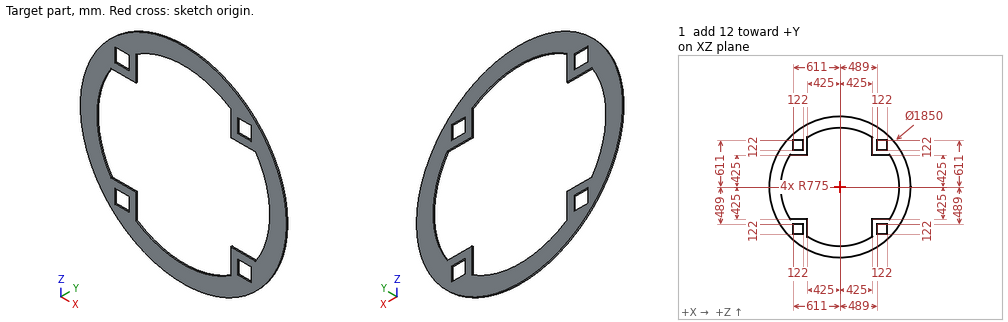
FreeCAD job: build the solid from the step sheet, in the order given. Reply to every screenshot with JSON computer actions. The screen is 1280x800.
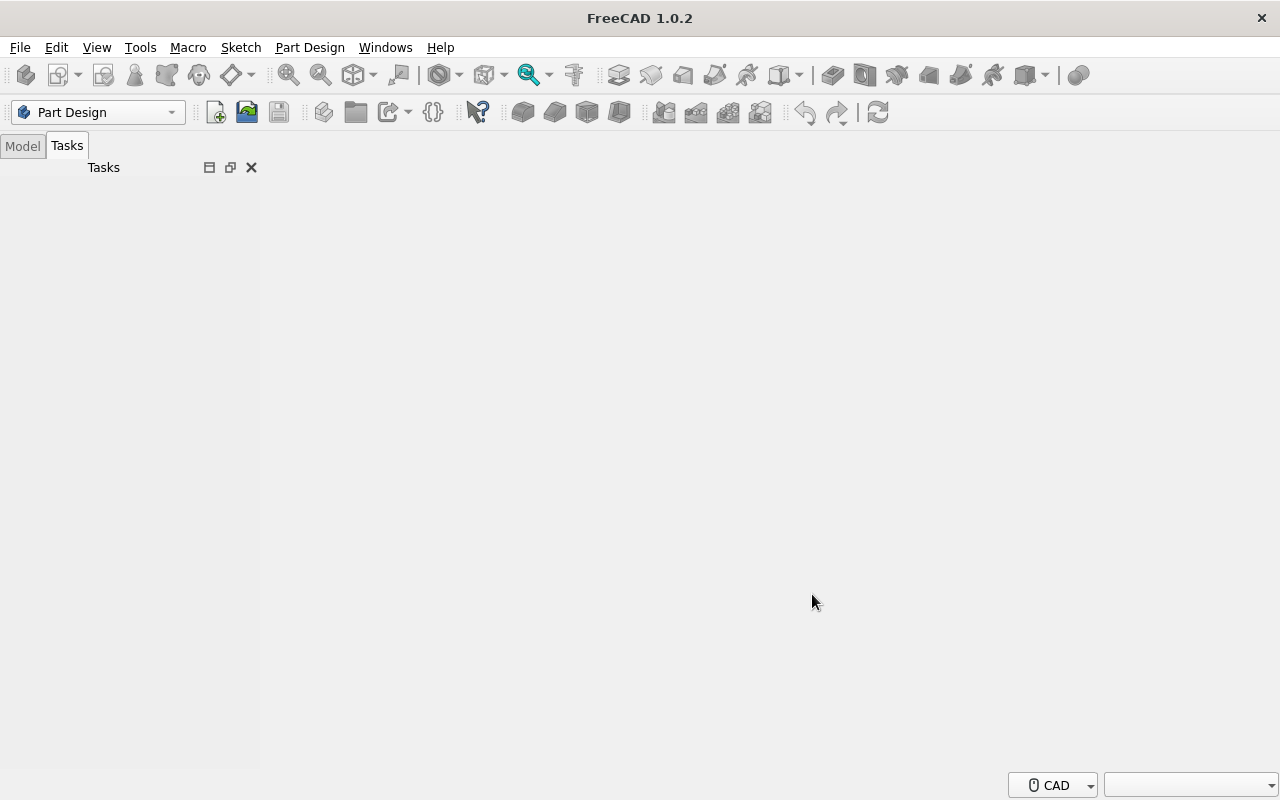
{"action": "left_click", "coordinate": [216, 112]}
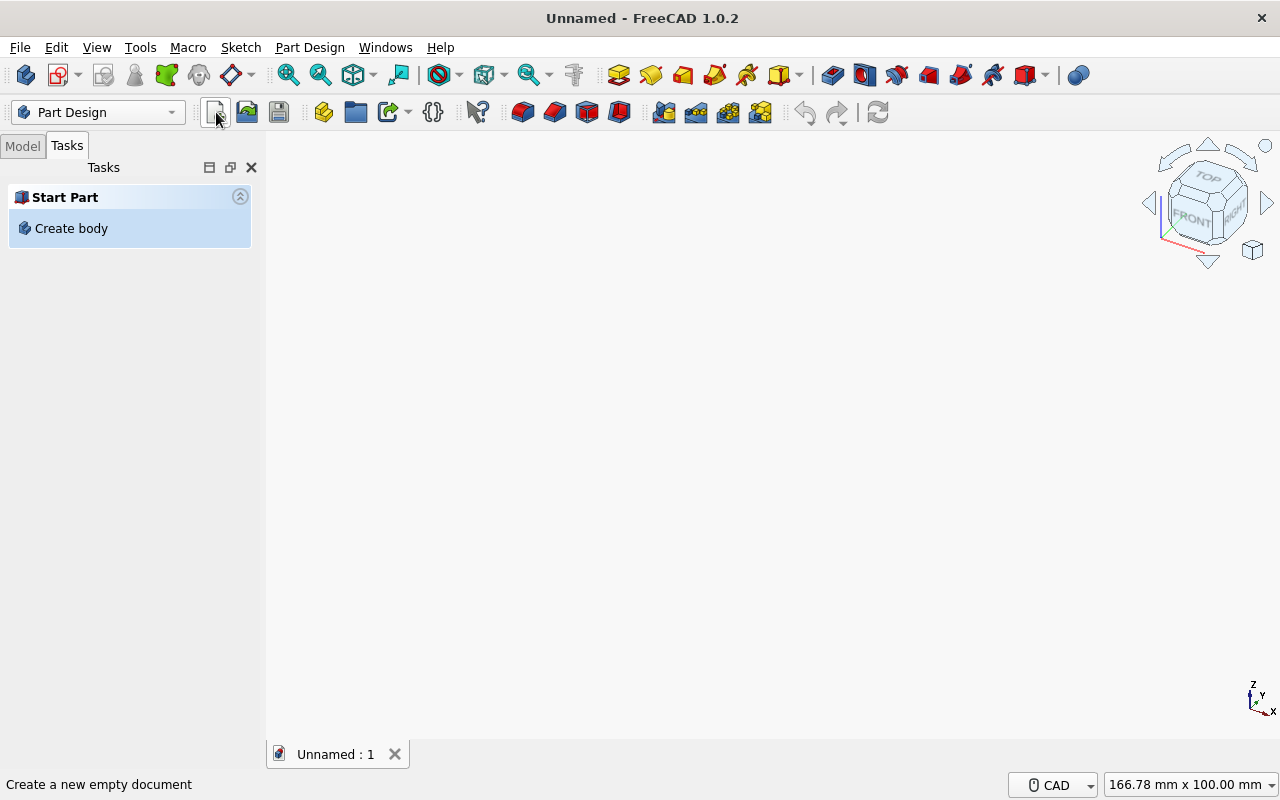
{"action": "left_click", "coordinate": [58, 76]}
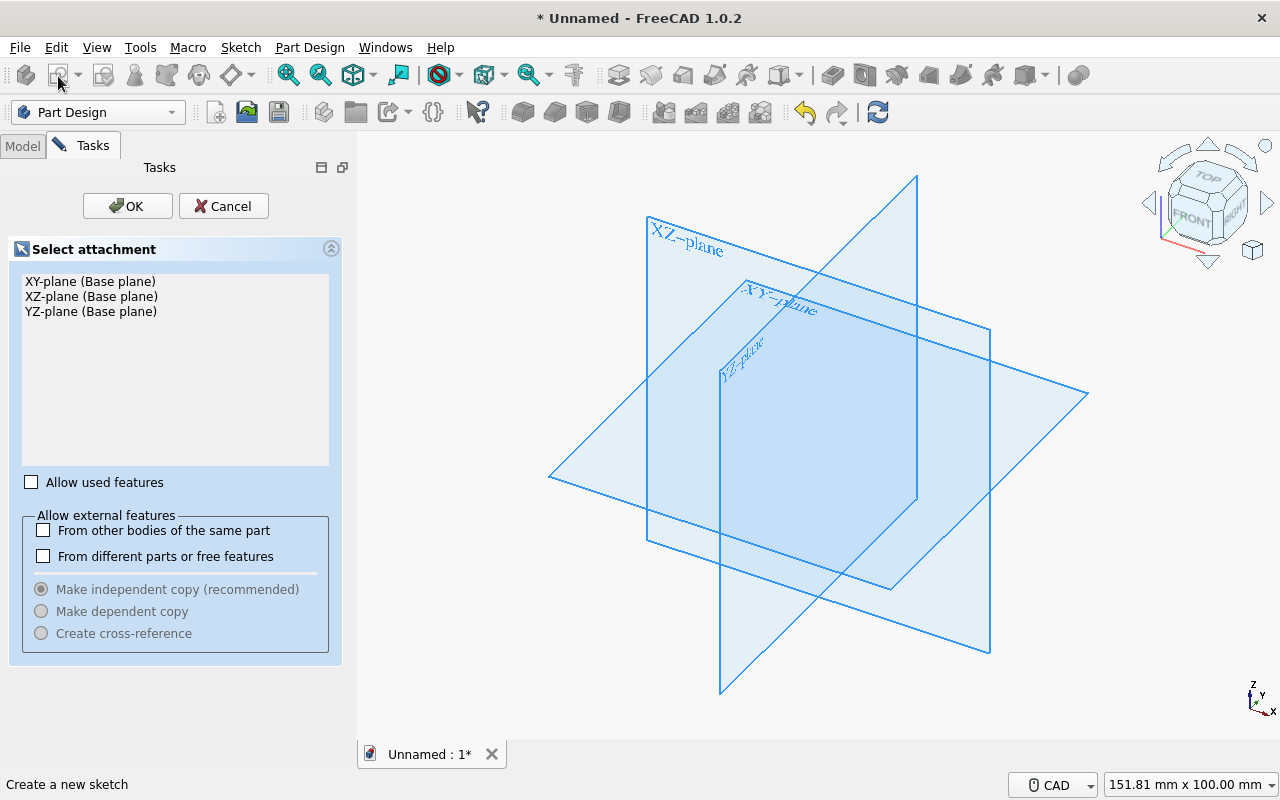
{"action": "left_click", "coordinate": [82, 296]}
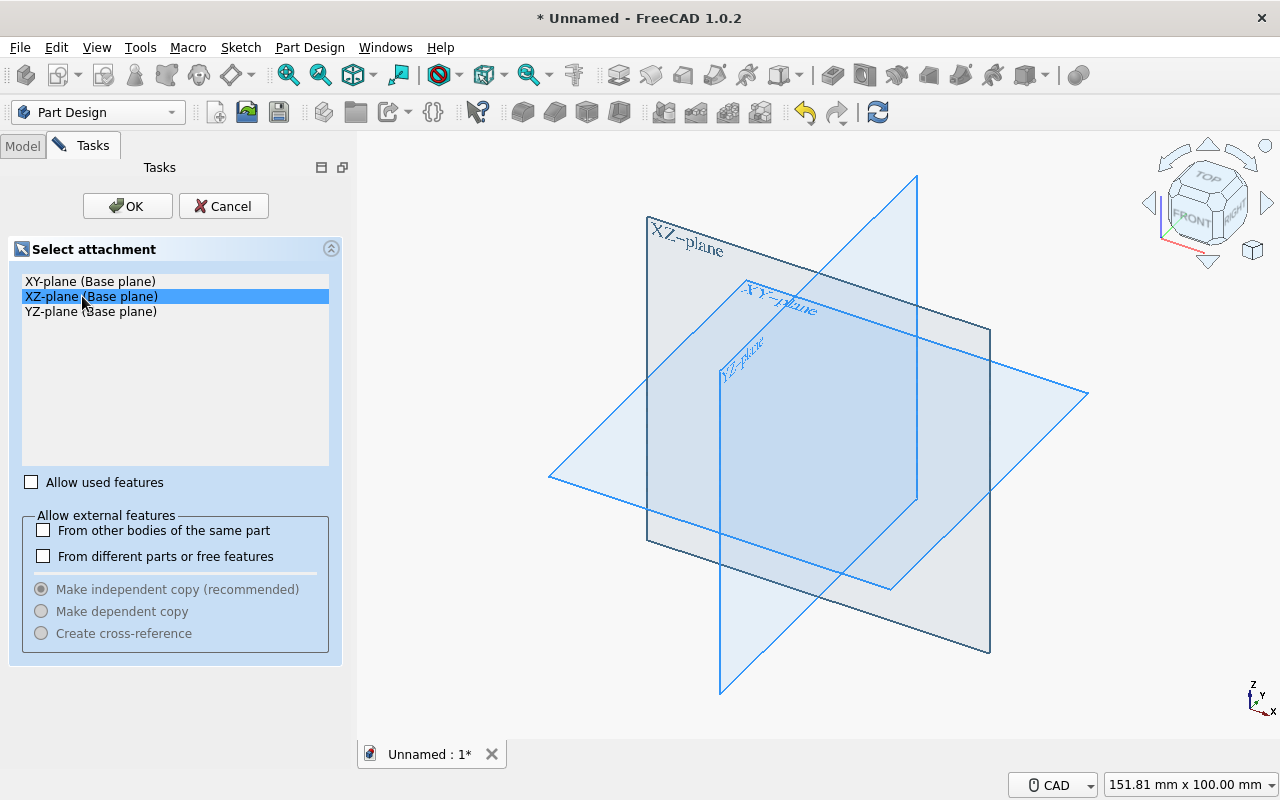
{"action": "left_click", "coordinate": [128, 206]}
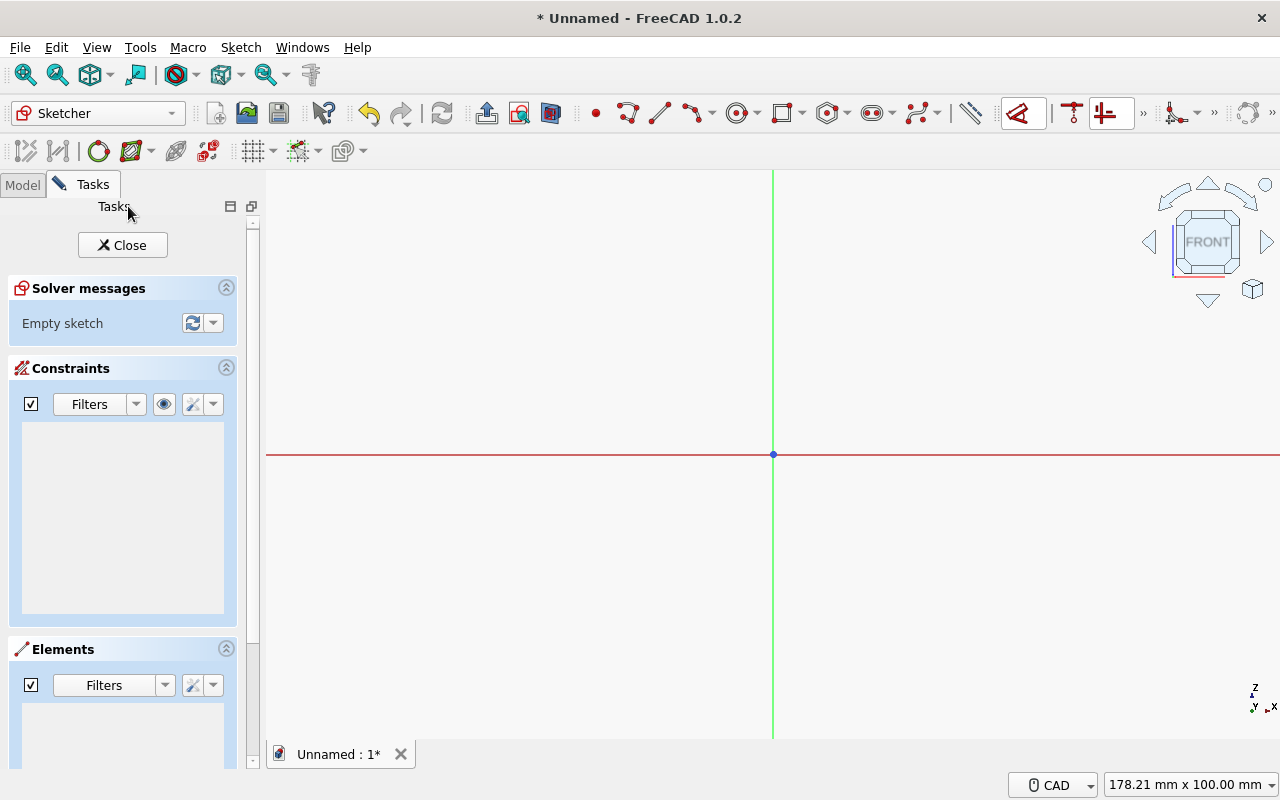
{"action": "scroll", "coordinate": [702, 454], "scroll_direction": "down", "scroll_amount": 16}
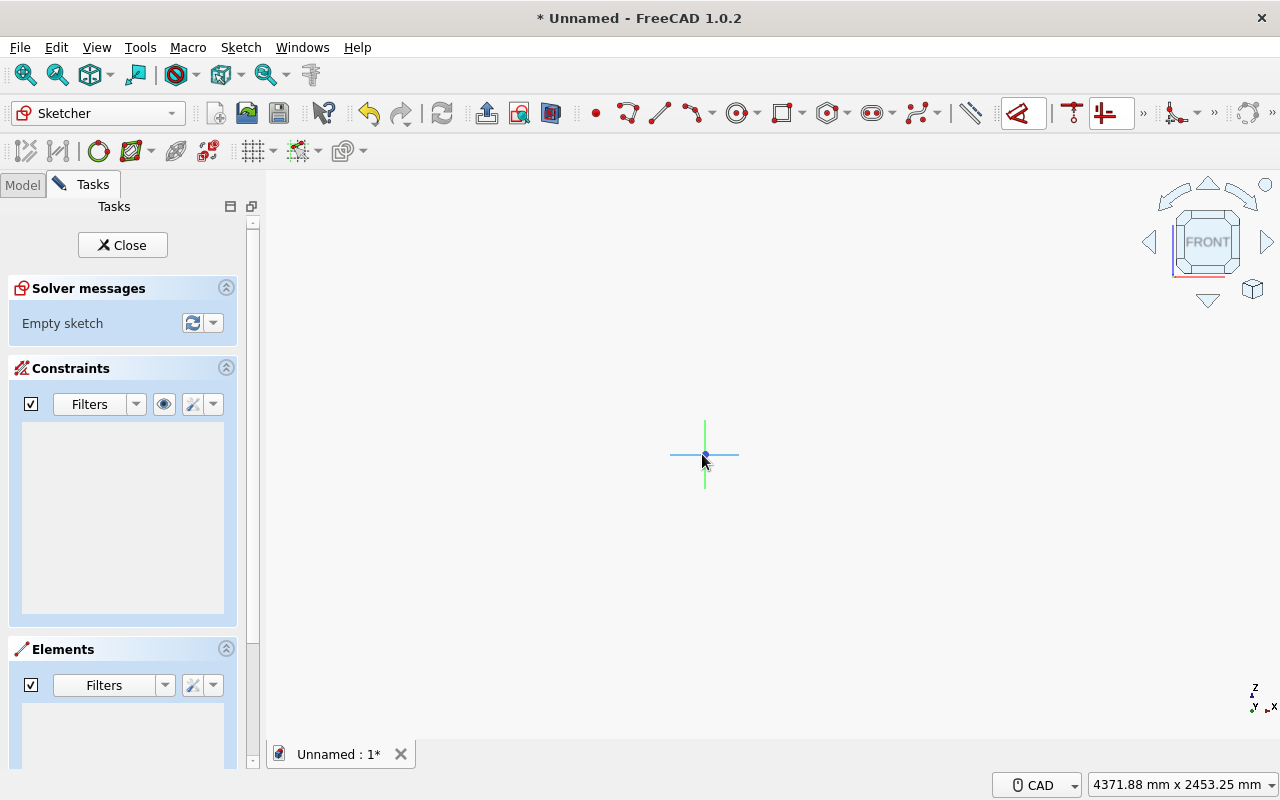
{"action": "left_click", "coordinate": [782, 114]}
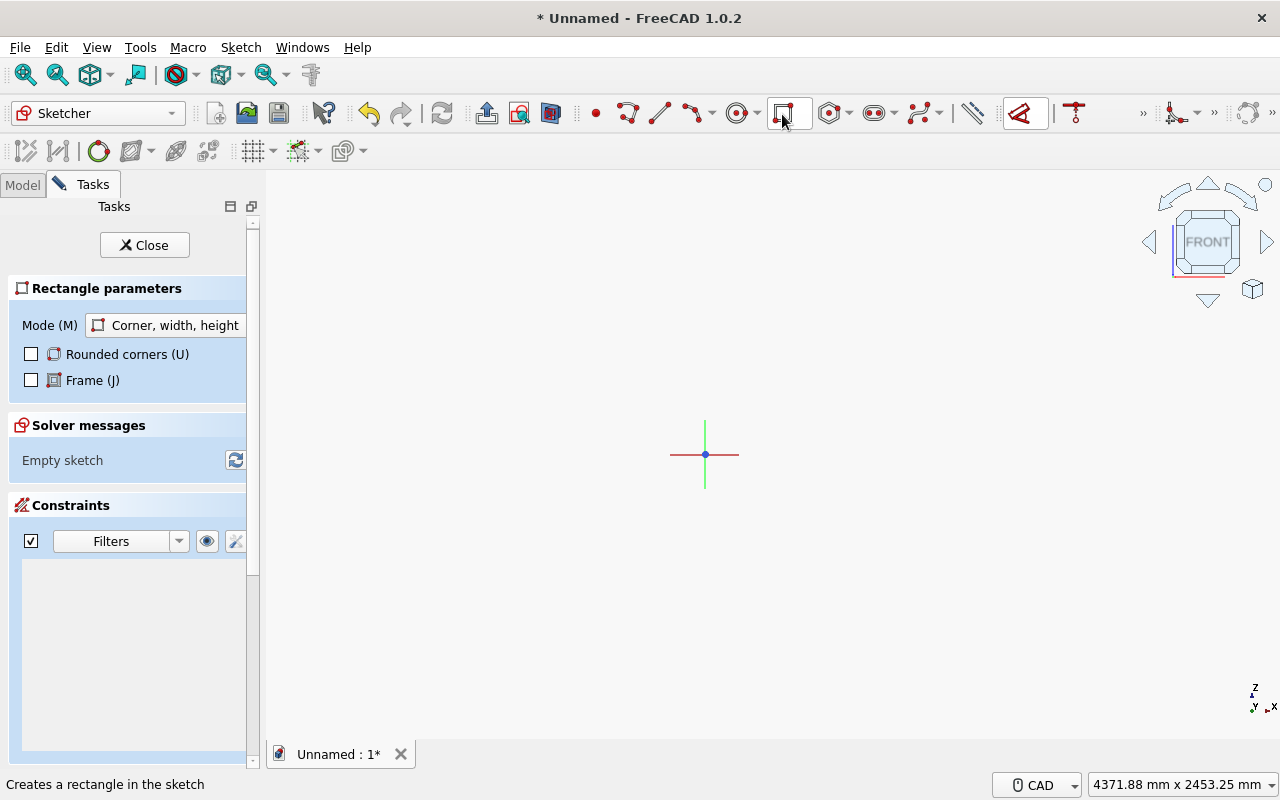
{"action": "left_click", "coordinate": [564, 568]}
{"action": "left_click", "coordinate": [592, 596]}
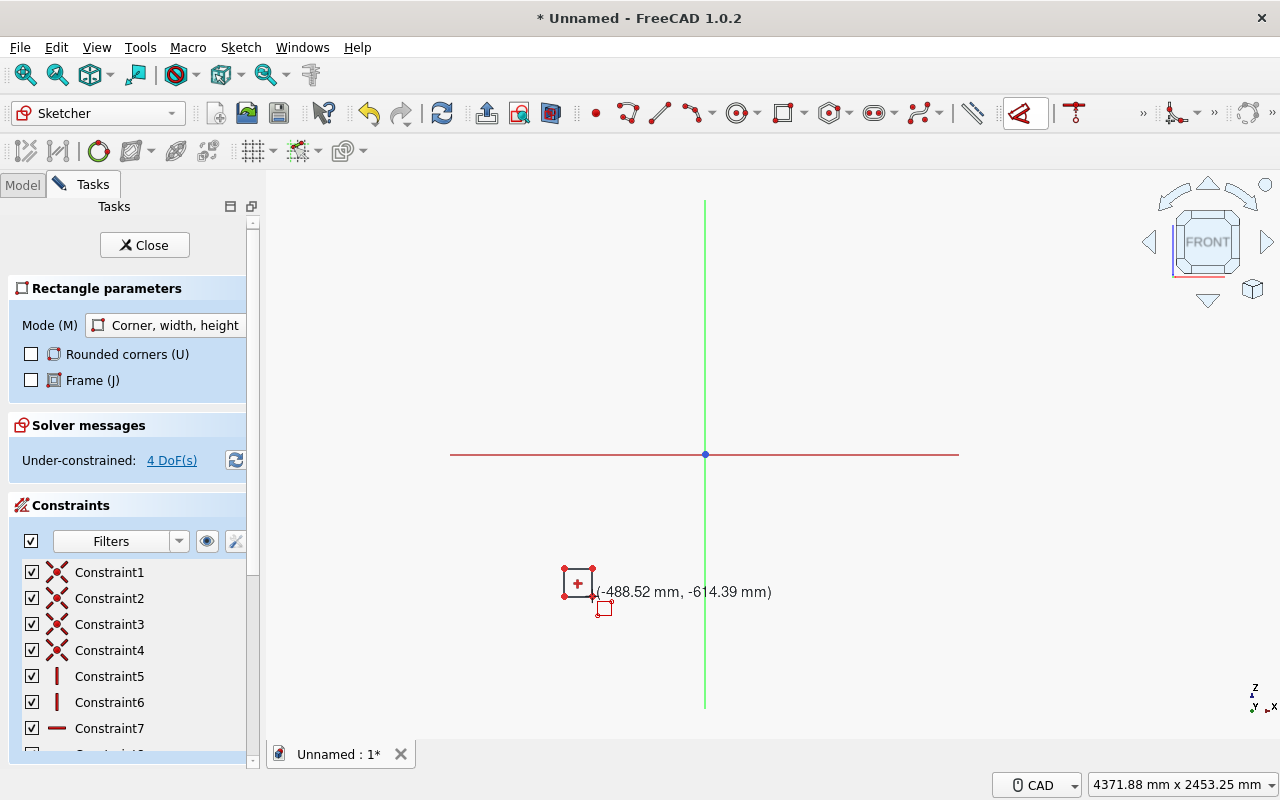
{"action": "left_click", "coordinate": [564, 313]}
{"action": "left_click", "coordinate": [592, 341]}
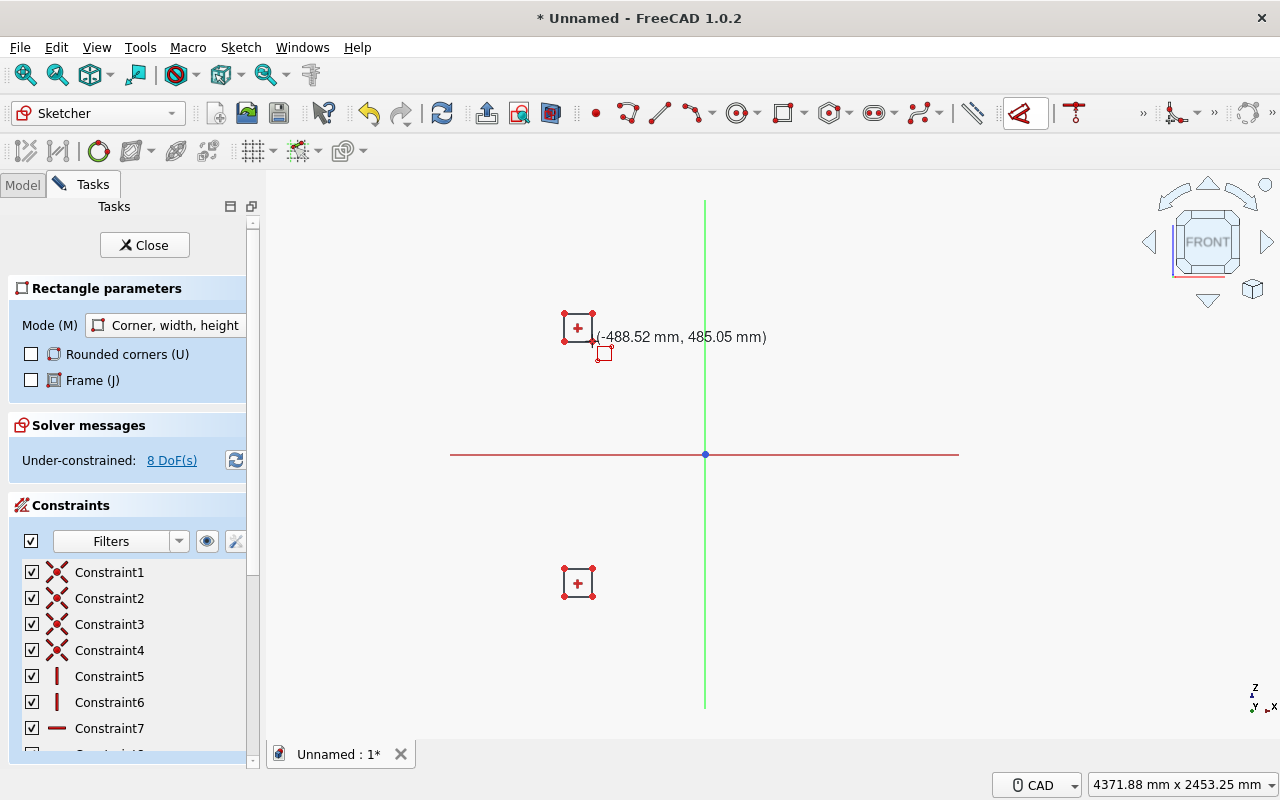
{"action": "left_click", "coordinate": [819, 568]}
{"action": "left_click", "coordinate": [847, 596]}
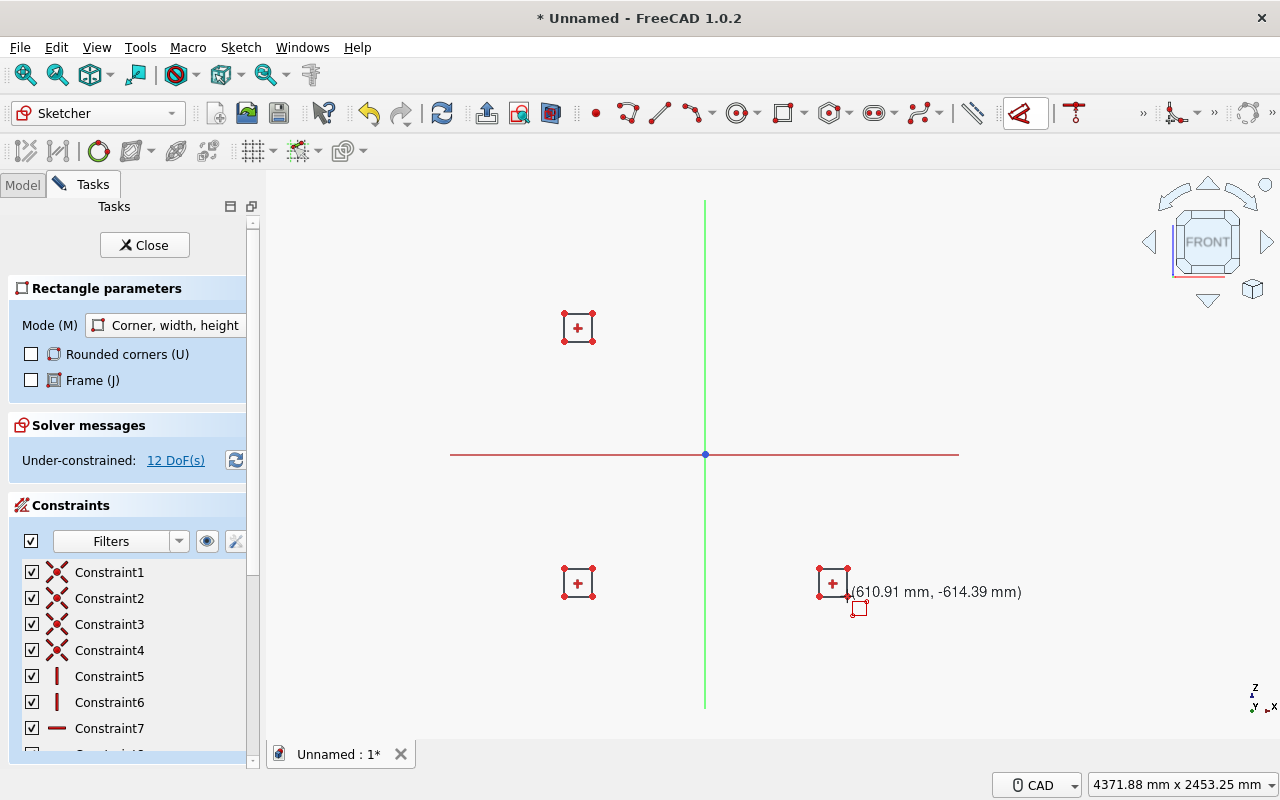
{"action": "key", "text": "g m"}